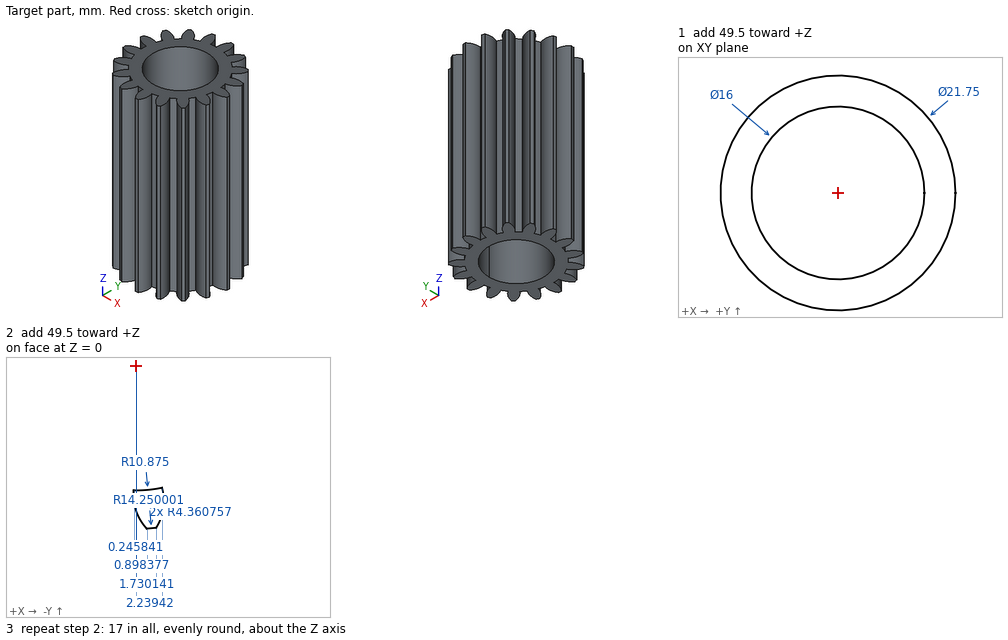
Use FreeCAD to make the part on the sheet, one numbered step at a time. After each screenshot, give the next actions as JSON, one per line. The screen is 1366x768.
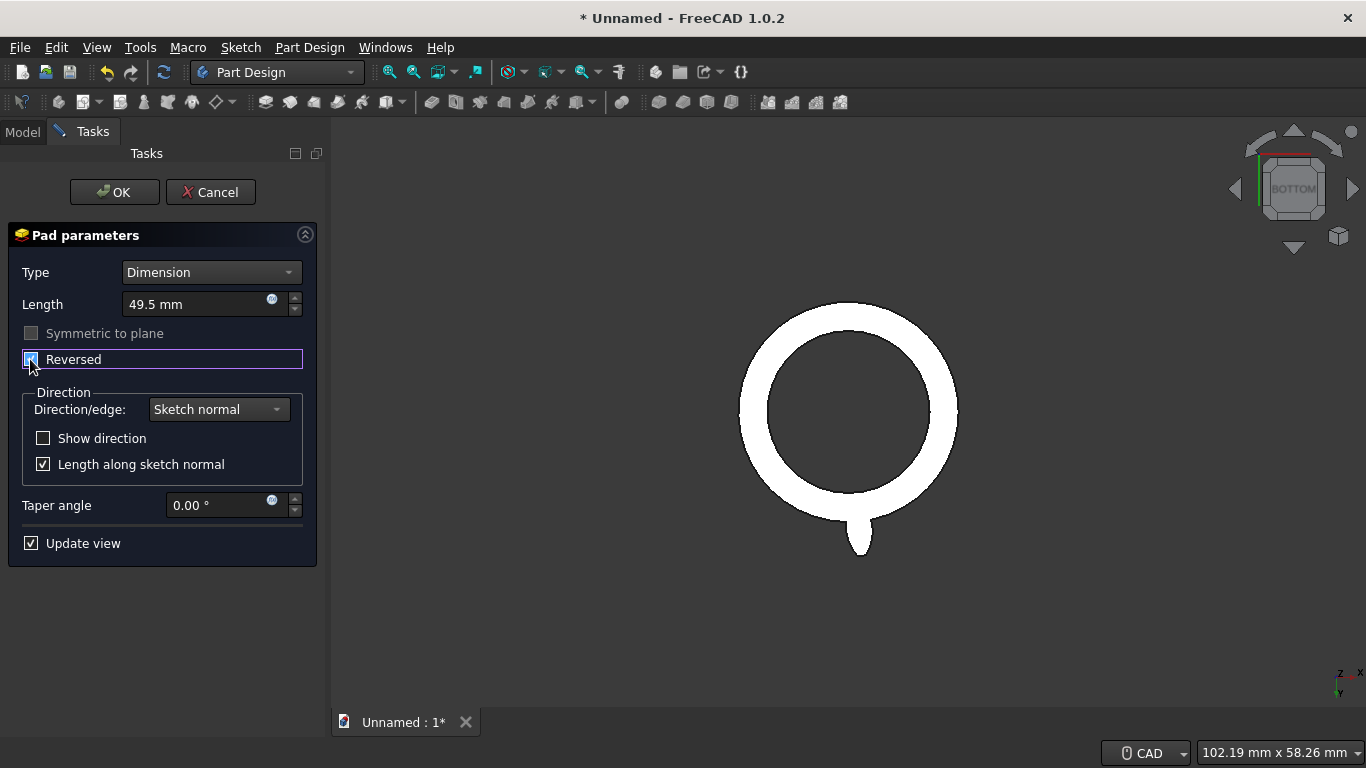
{"action": "left_click", "coordinate": [115, 192]}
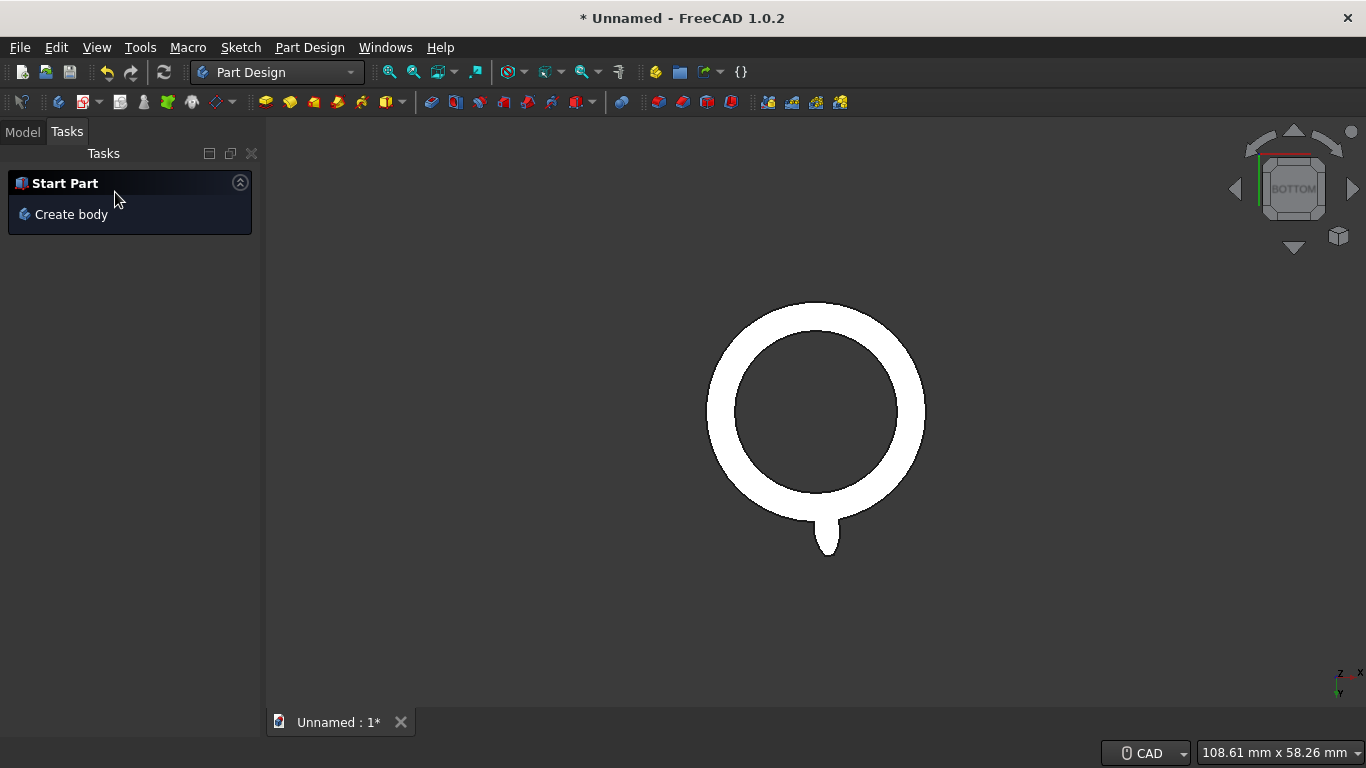
{"action": "left_click", "coordinate": [390, 72]}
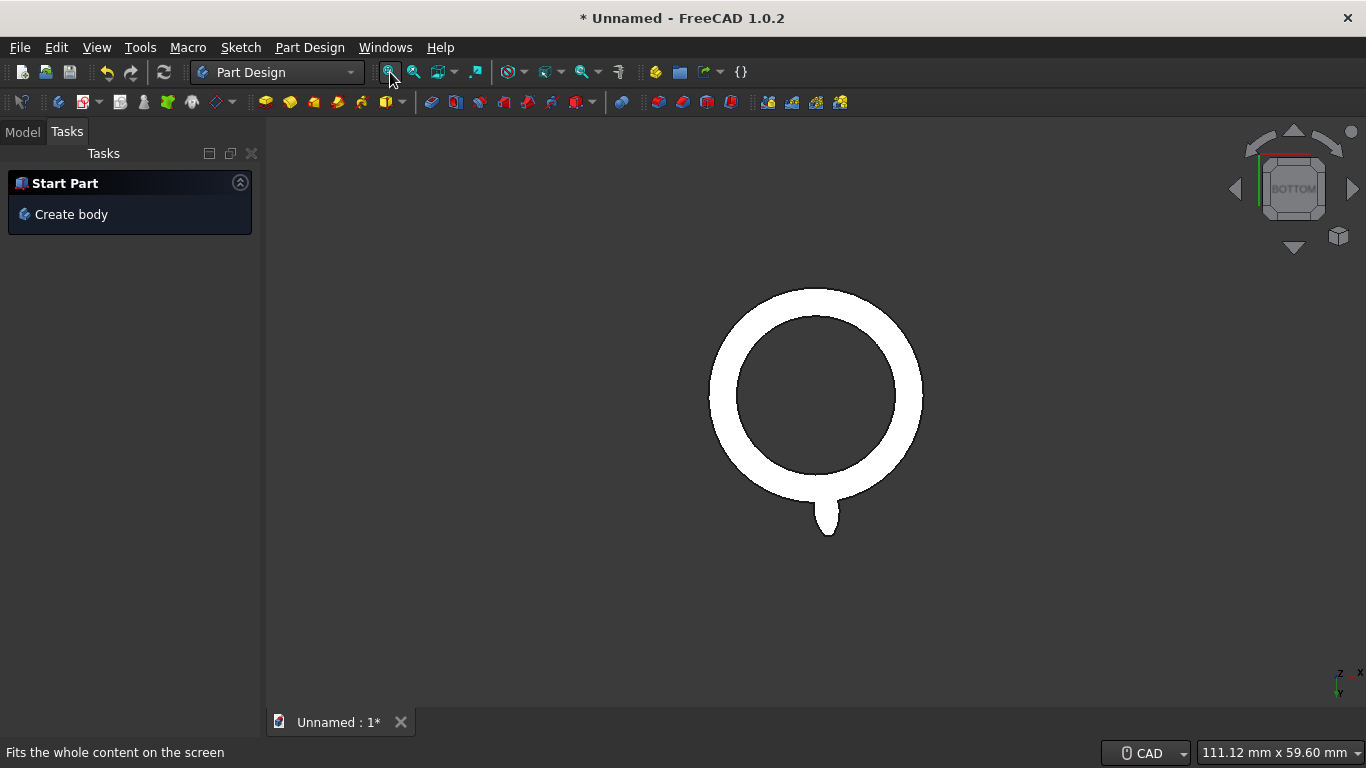
{"action": "left_click", "coordinate": [23, 131]}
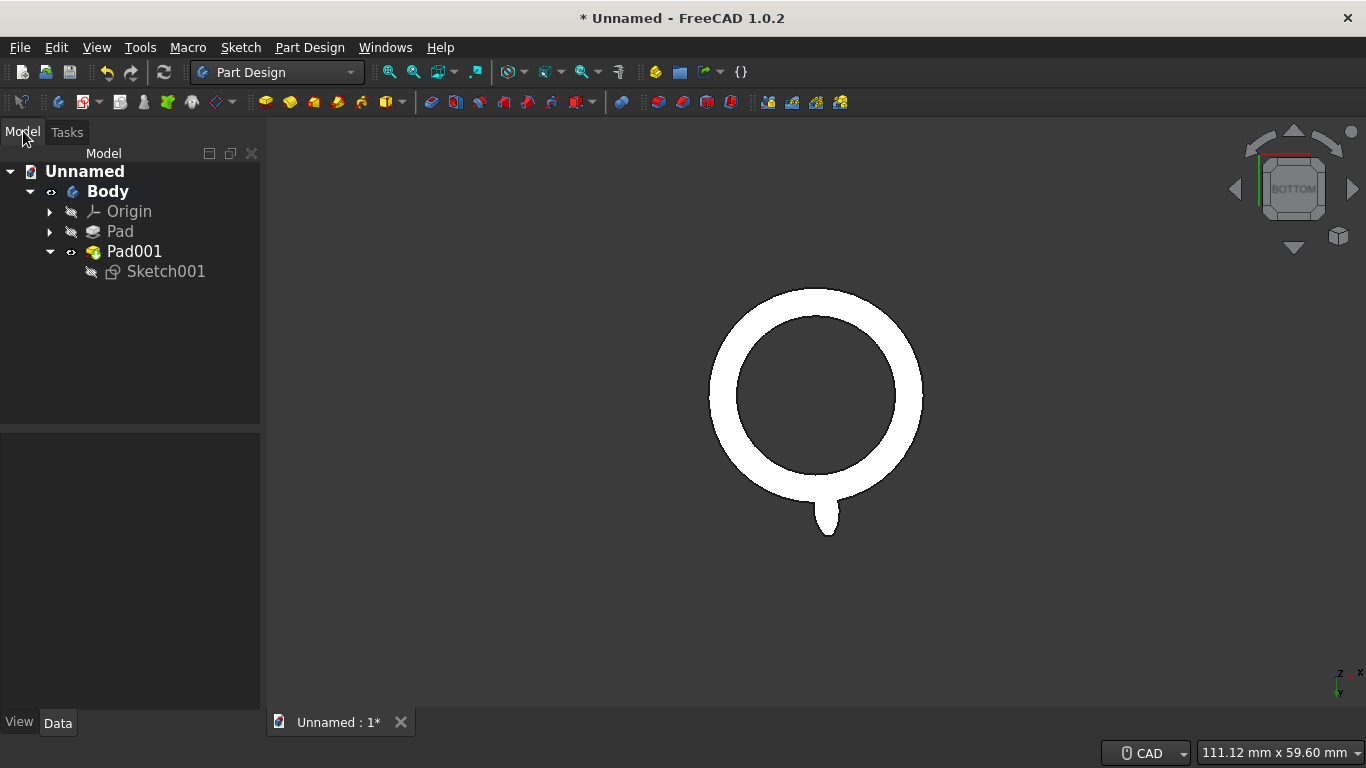
{"action": "left_click", "coordinate": [116, 252]}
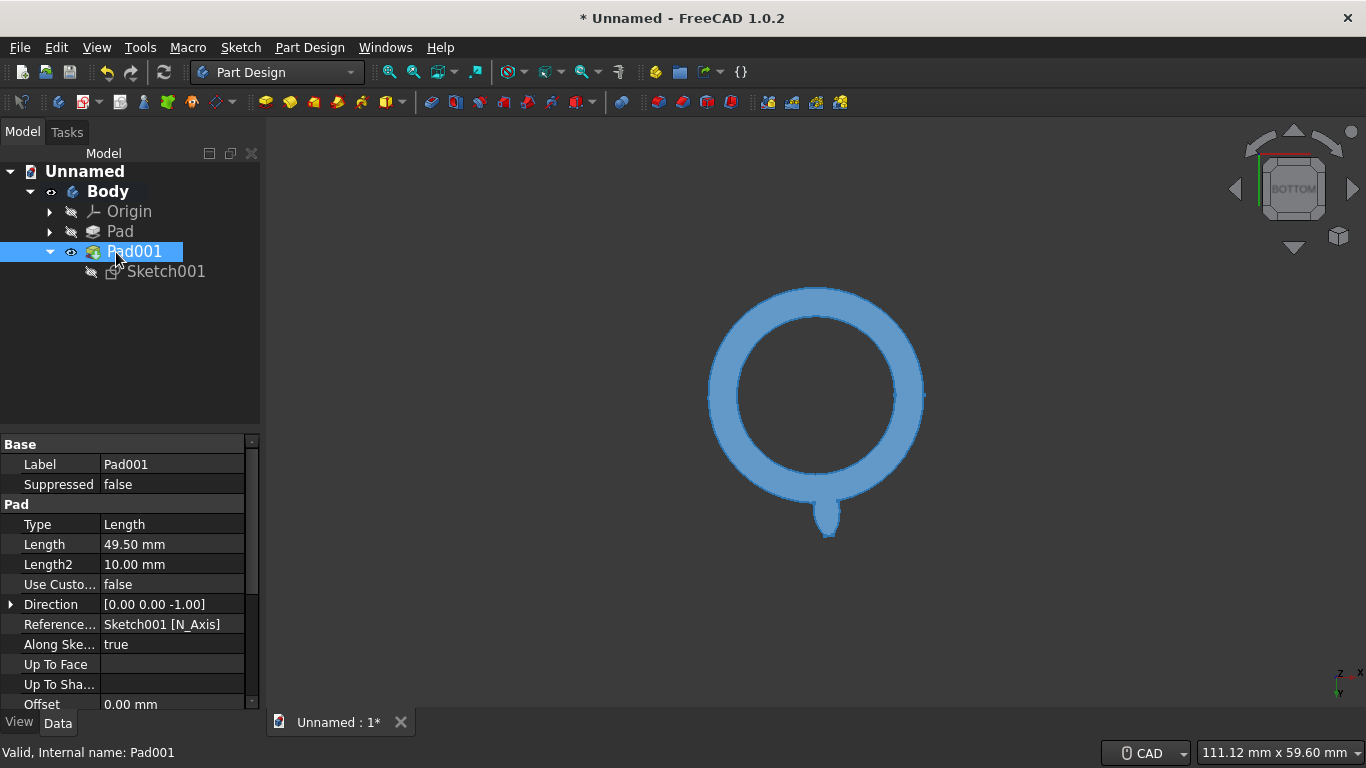
{"action": "left_click", "coordinate": [816, 102]}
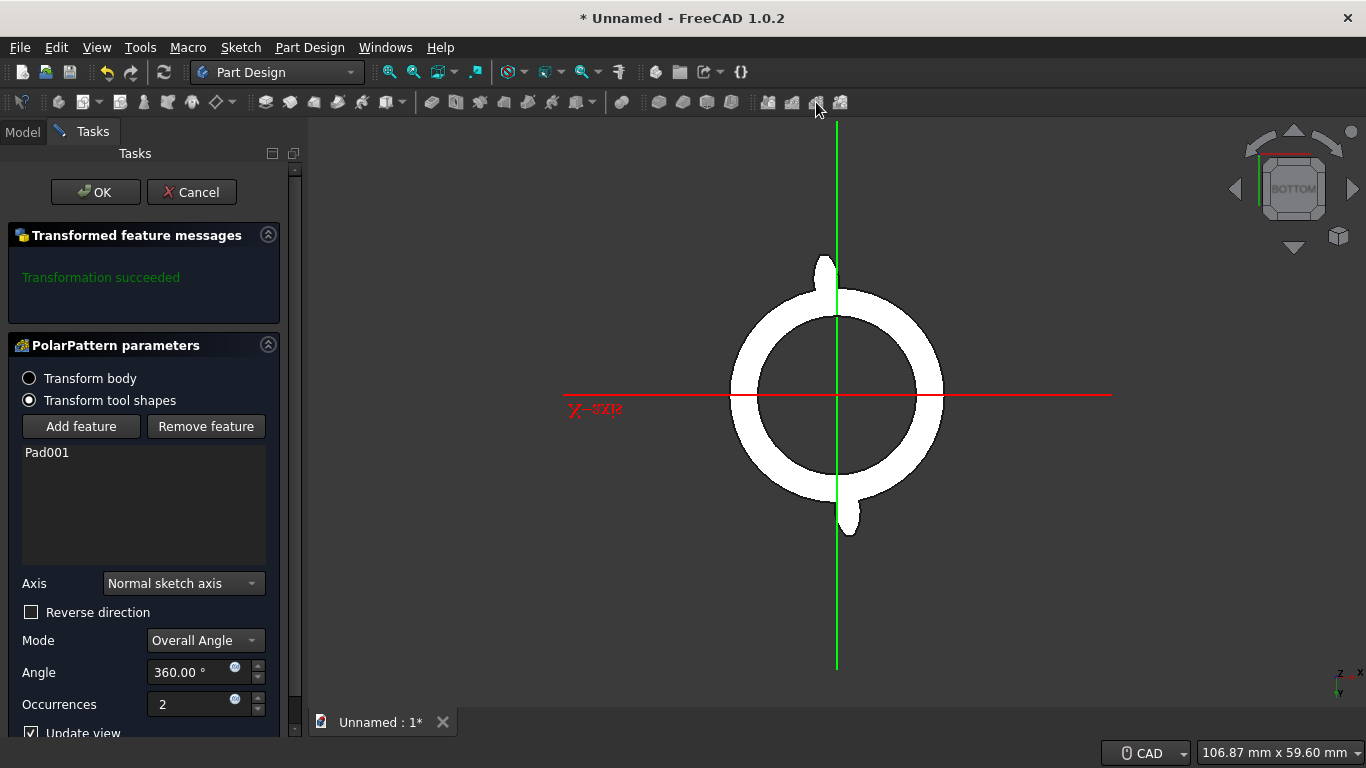
{"action": "left_click", "coordinate": [184, 584]}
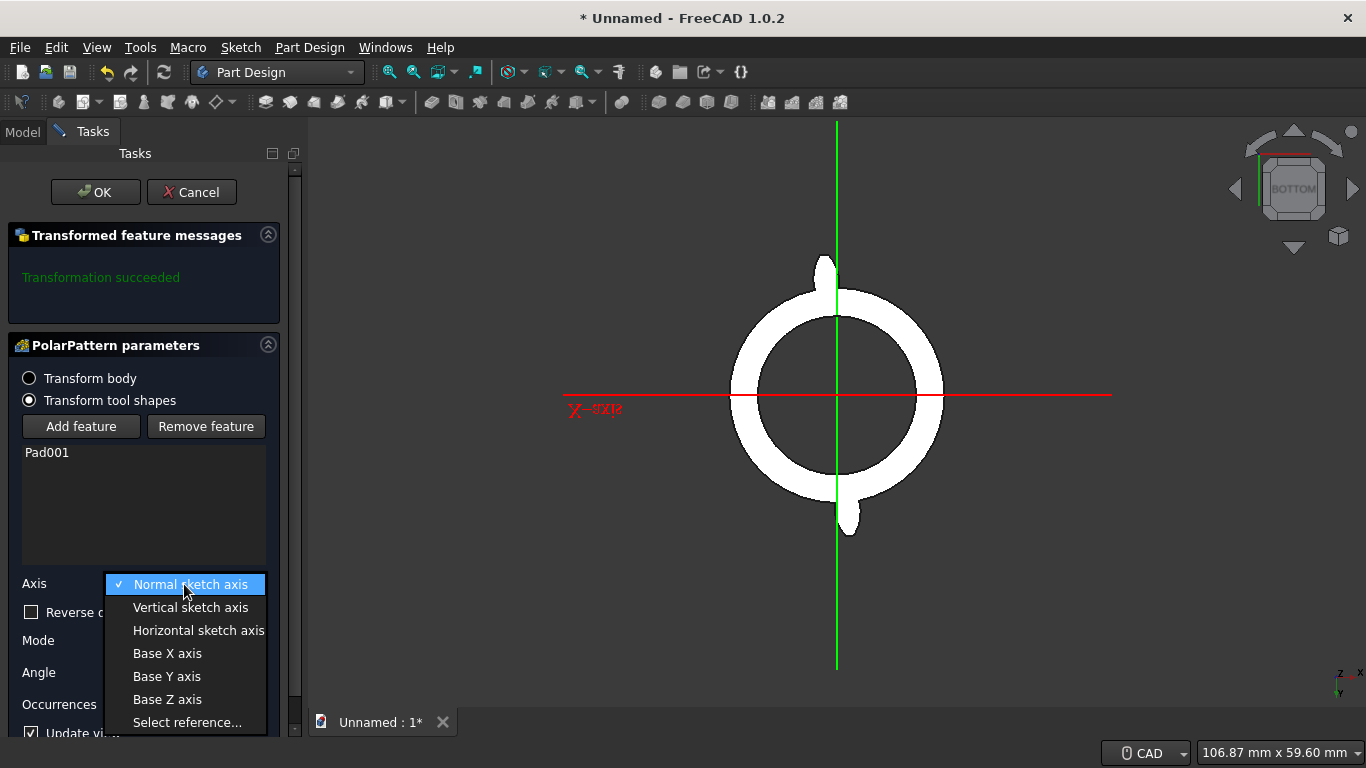
{"action": "left_click", "coordinate": [184, 700]}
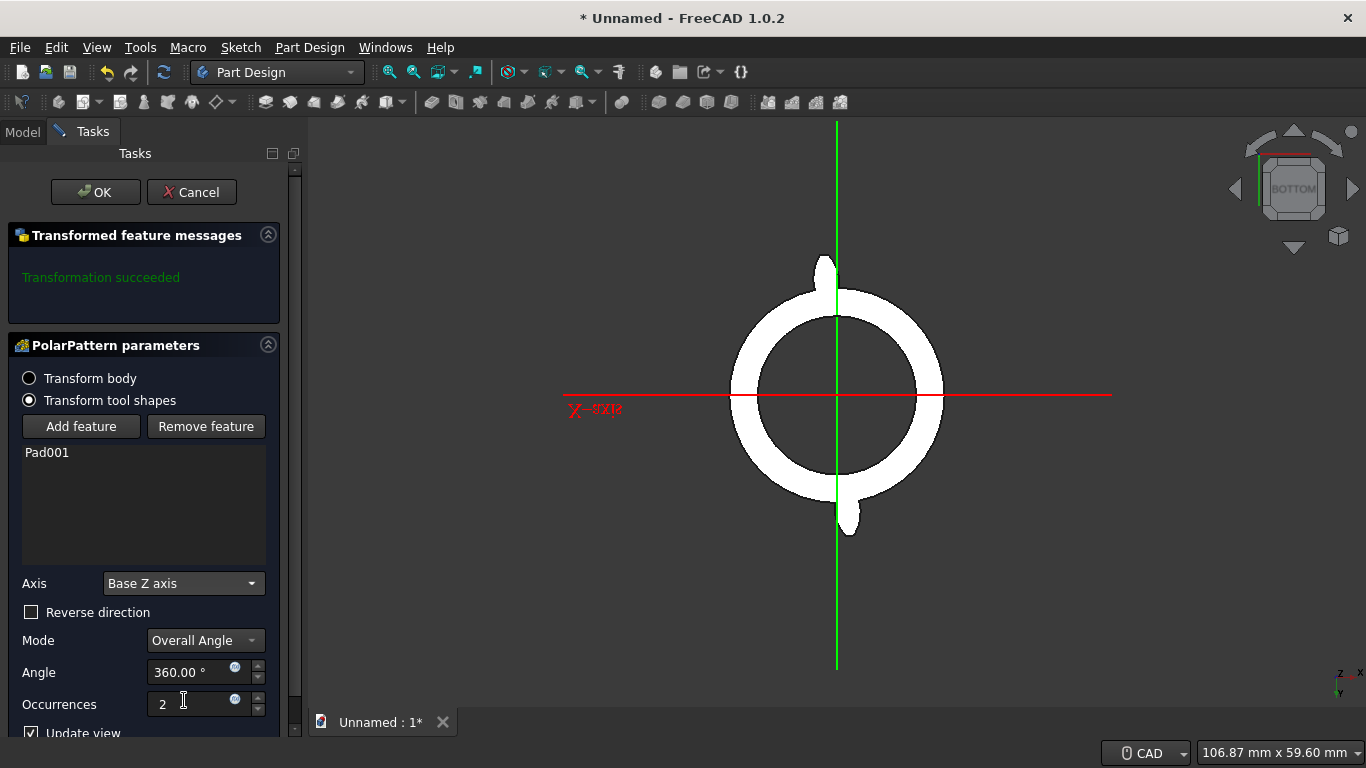
{"action": "triple_click", "coordinate": [198, 704]}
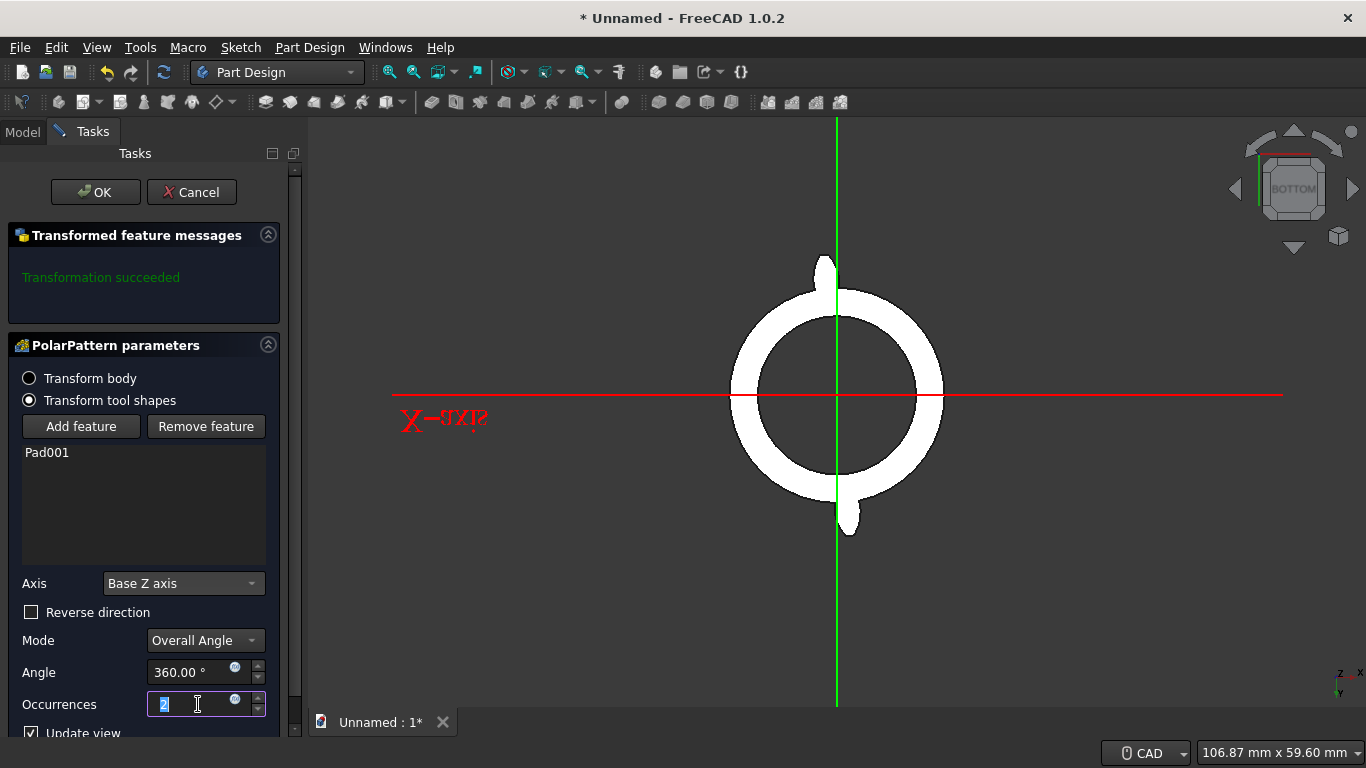
{"action": "type", "text": "17"}
{"action": "key", "text": "Tab"}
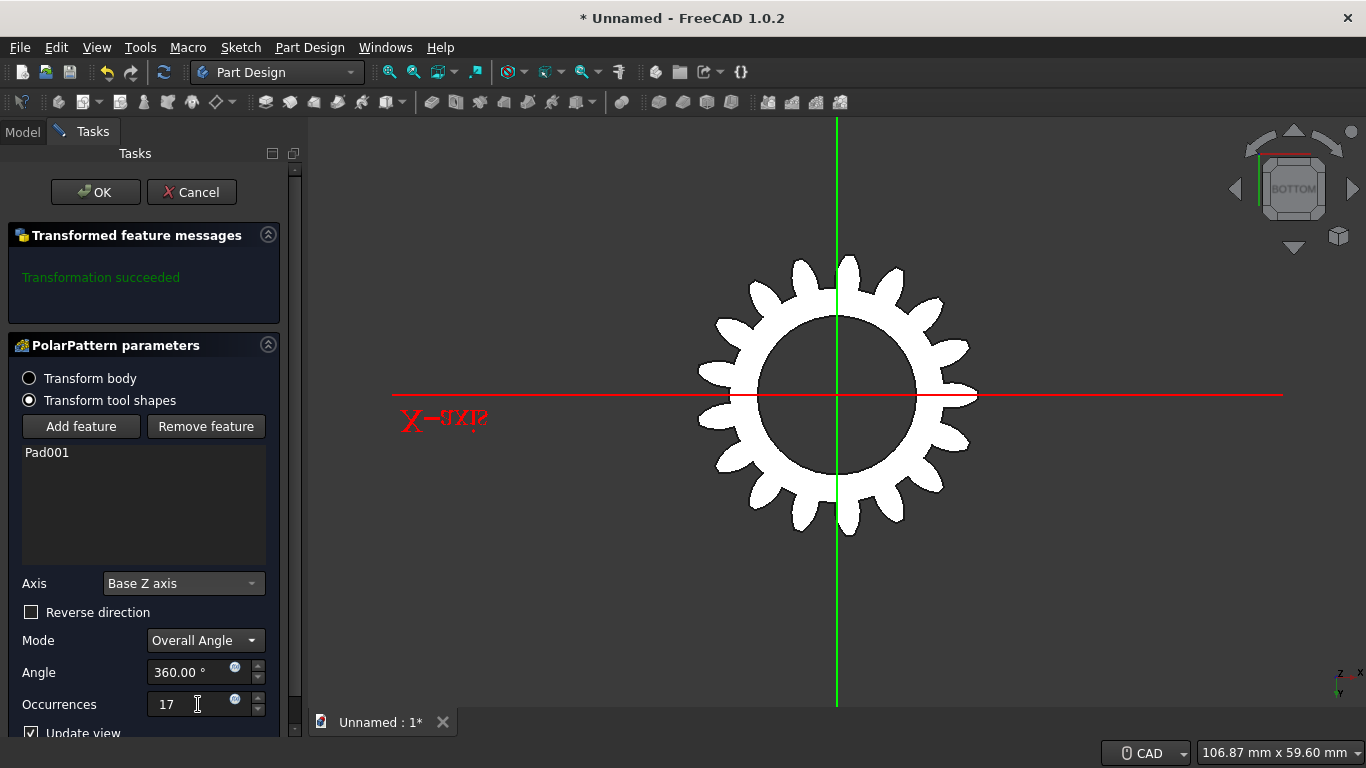
{"action": "left_click", "coordinate": [96, 192]}